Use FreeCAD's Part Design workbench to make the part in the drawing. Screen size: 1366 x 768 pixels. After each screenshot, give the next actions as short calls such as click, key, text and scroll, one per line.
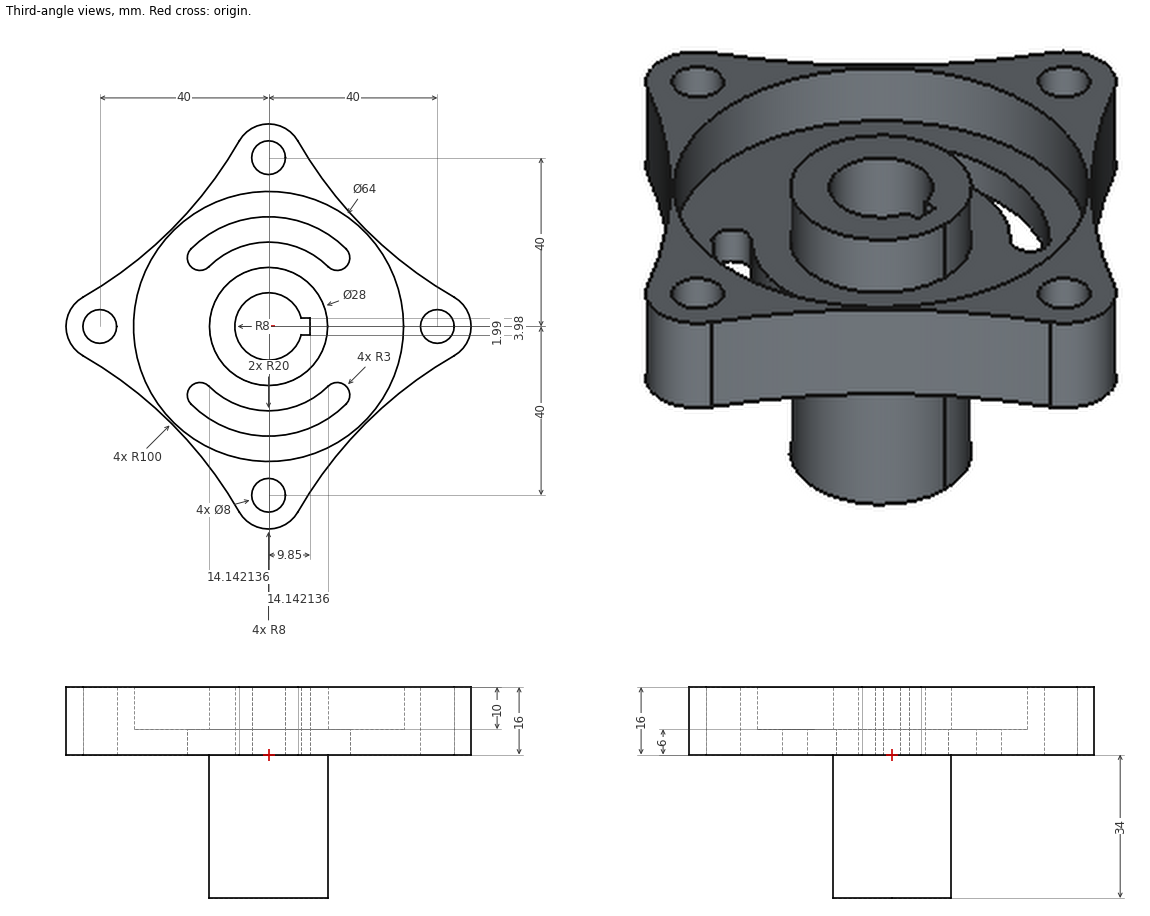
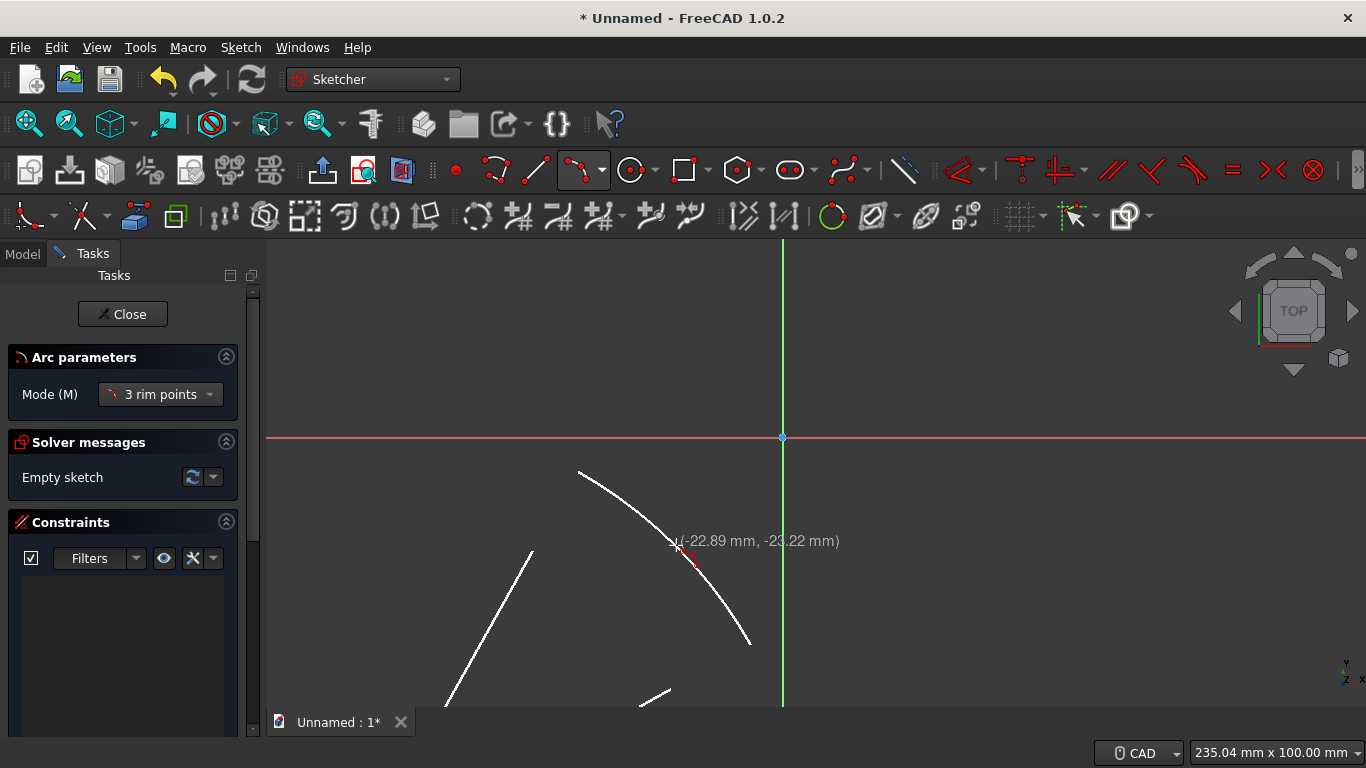
click(675, 545)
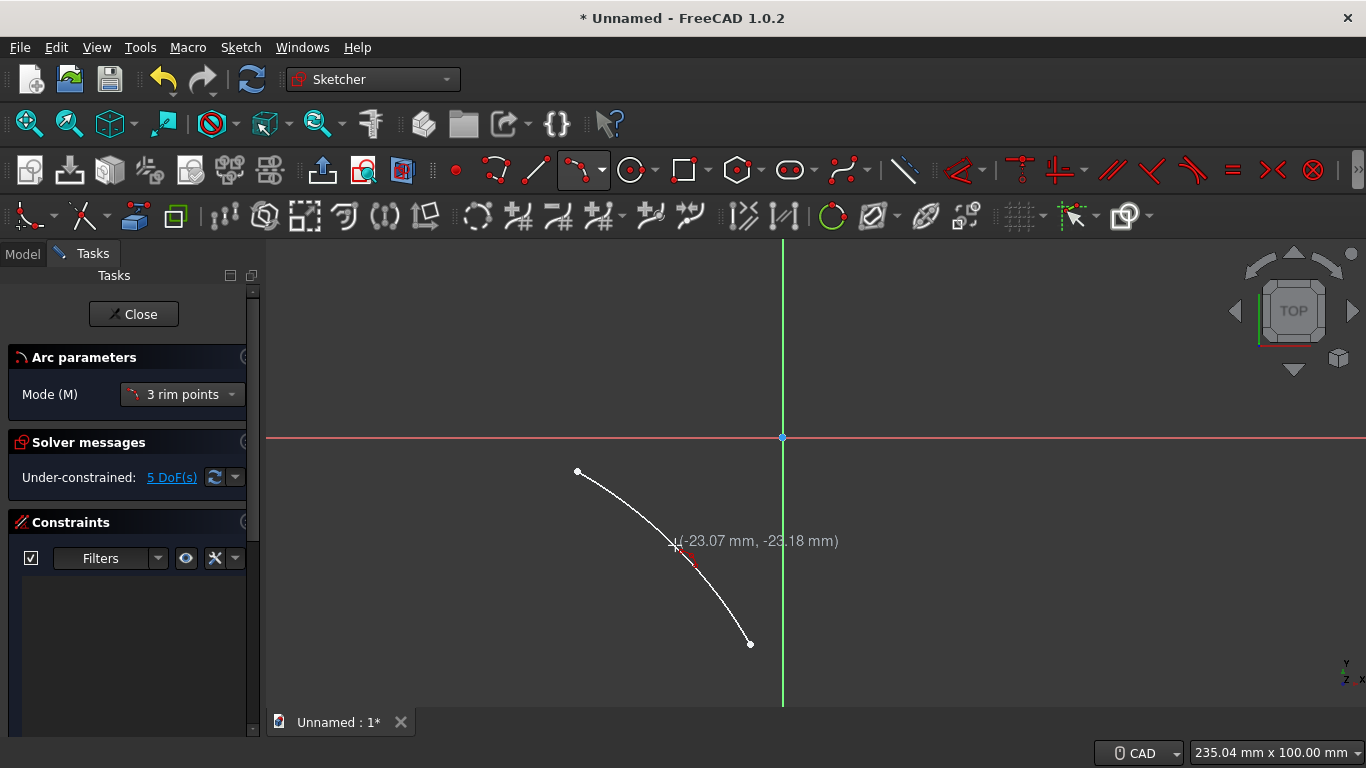
click(750, 645)
click(815, 643)
click(798, 659)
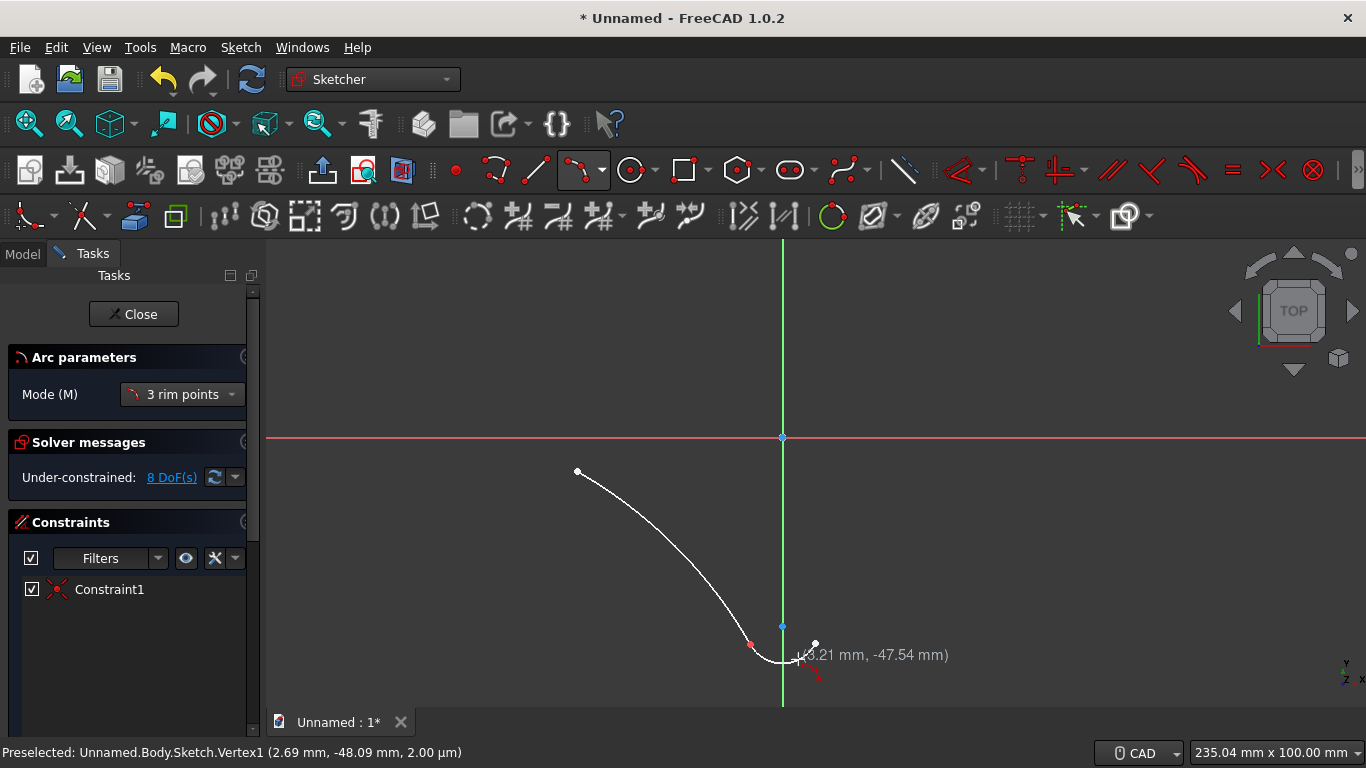
click(815, 644)
click(989, 470)
click(891, 545)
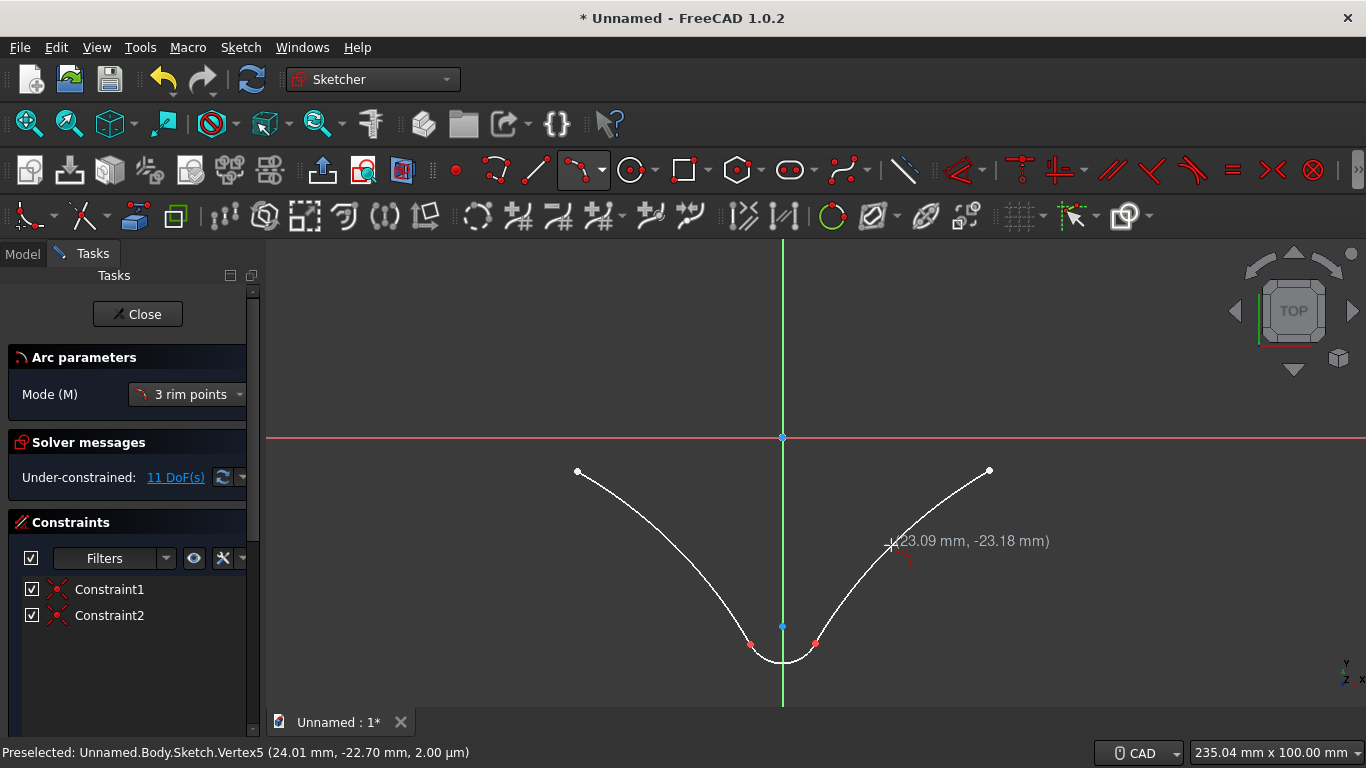
click(989, 471)
click(989, 405)
click(1004, 453)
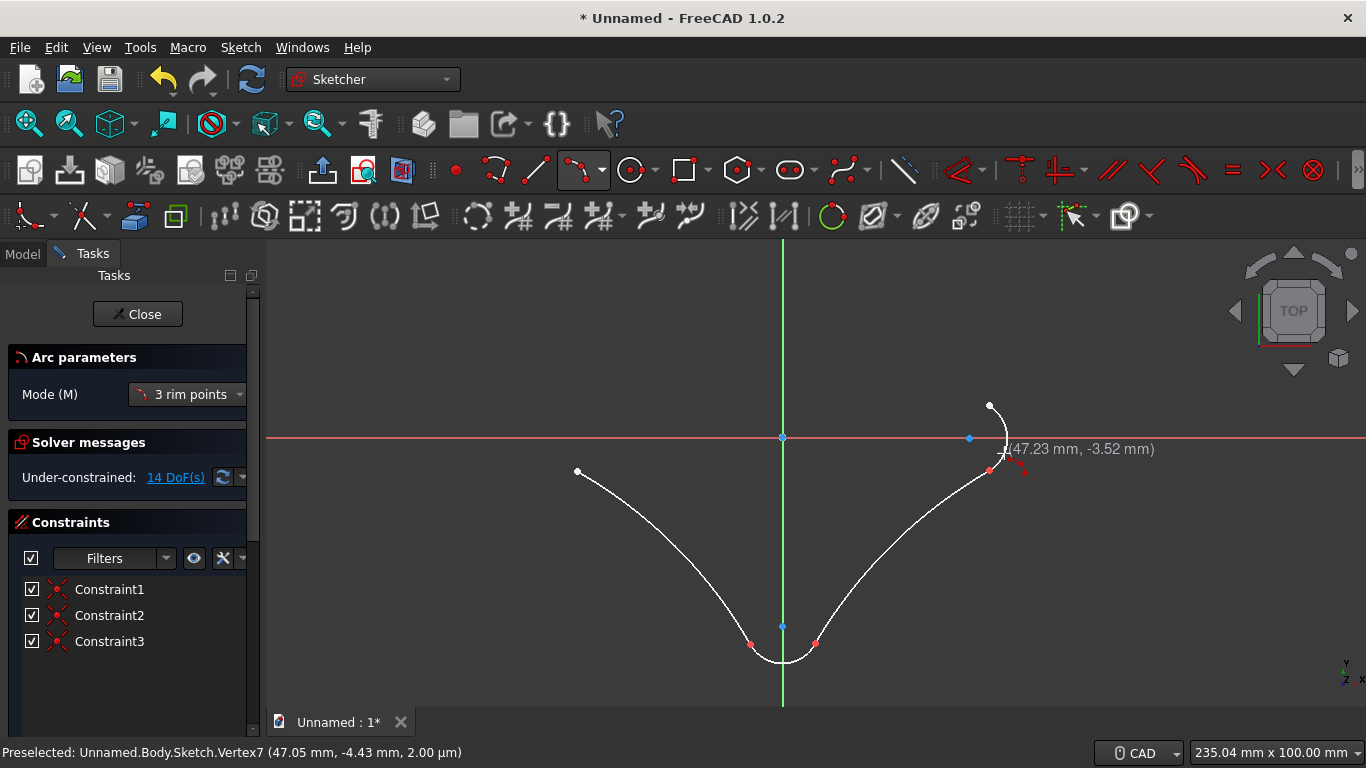
click(989, 406)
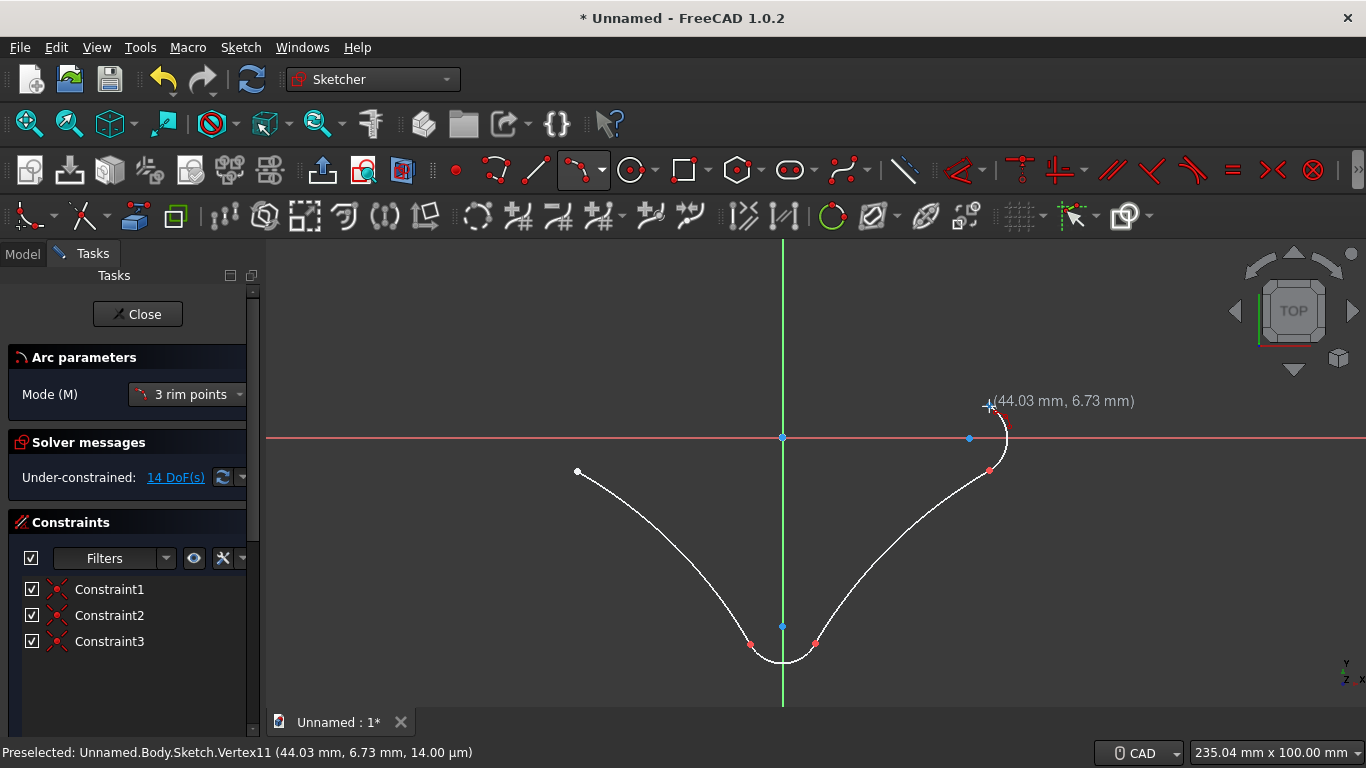
scroll(675, 545, down, 2)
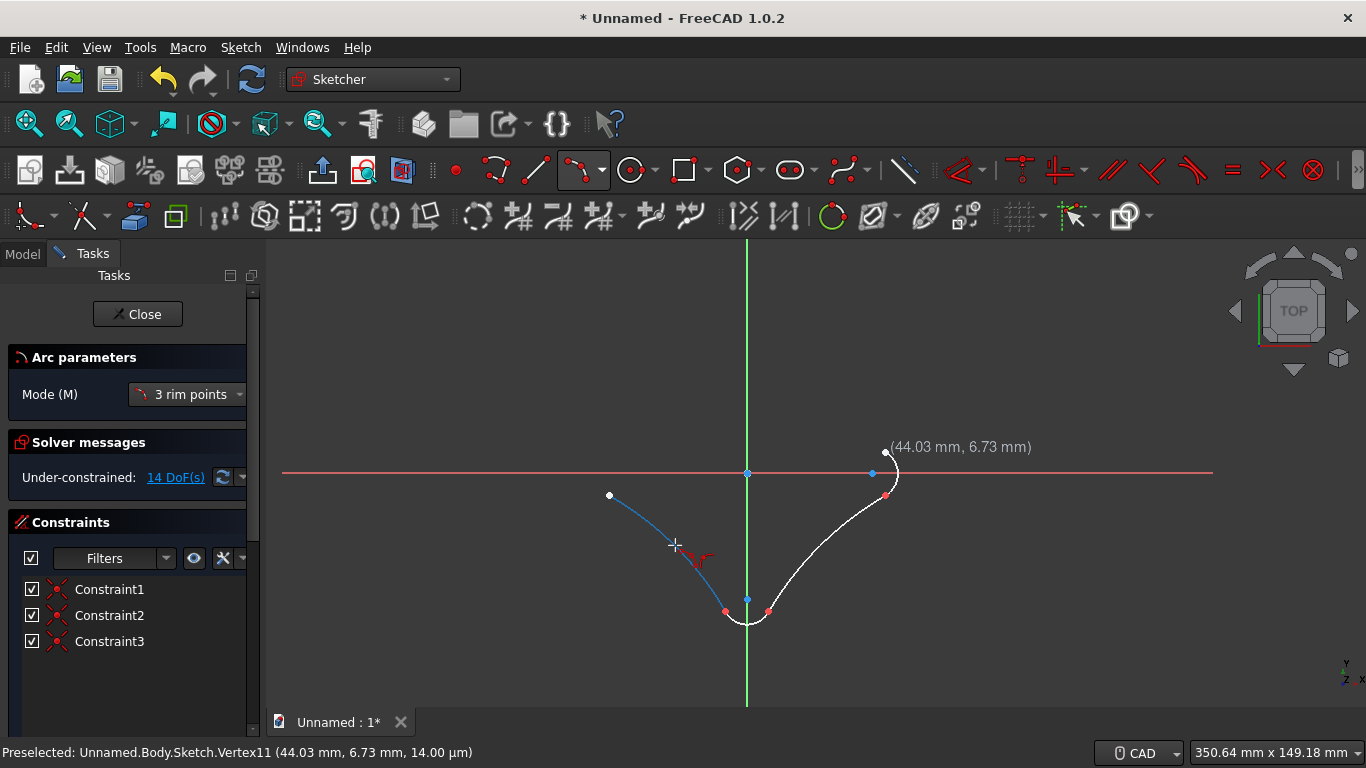
click(769, 335)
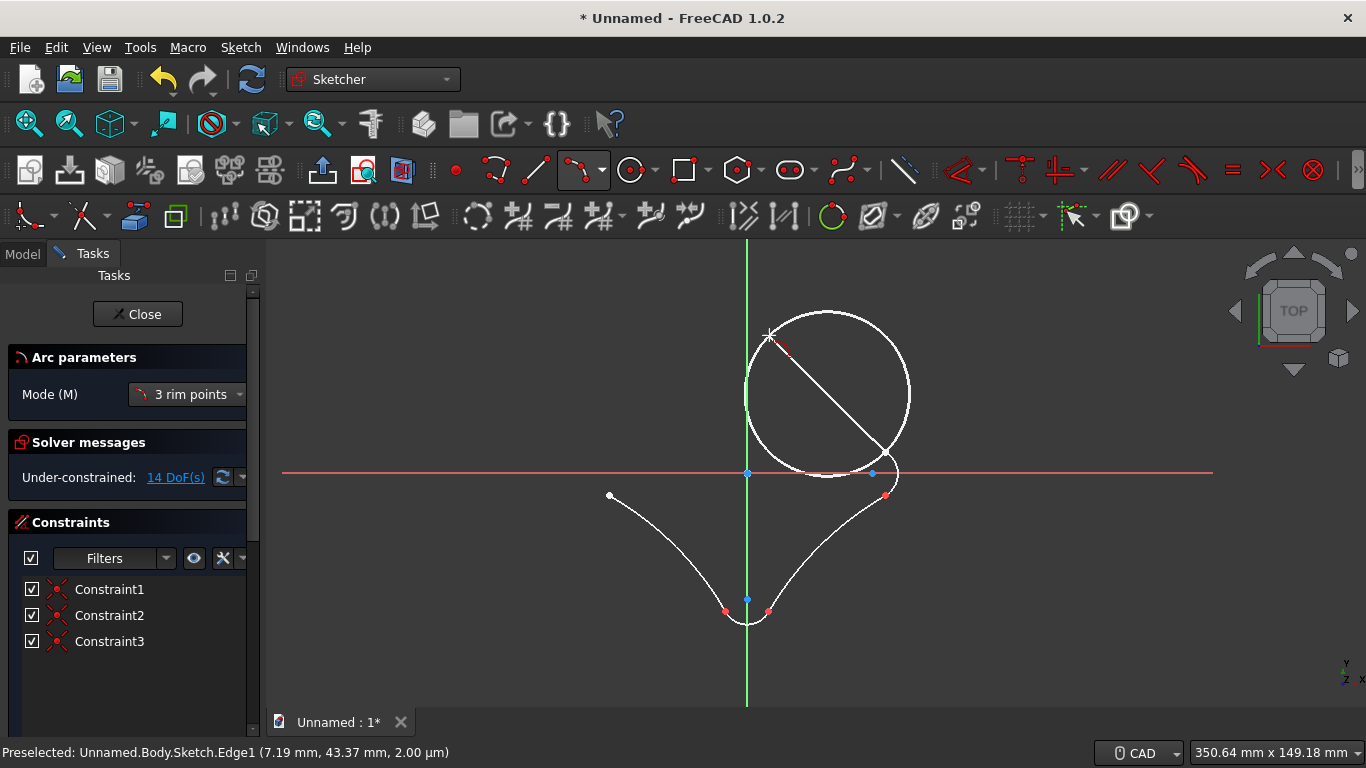
scroll(820, 401, up, 2)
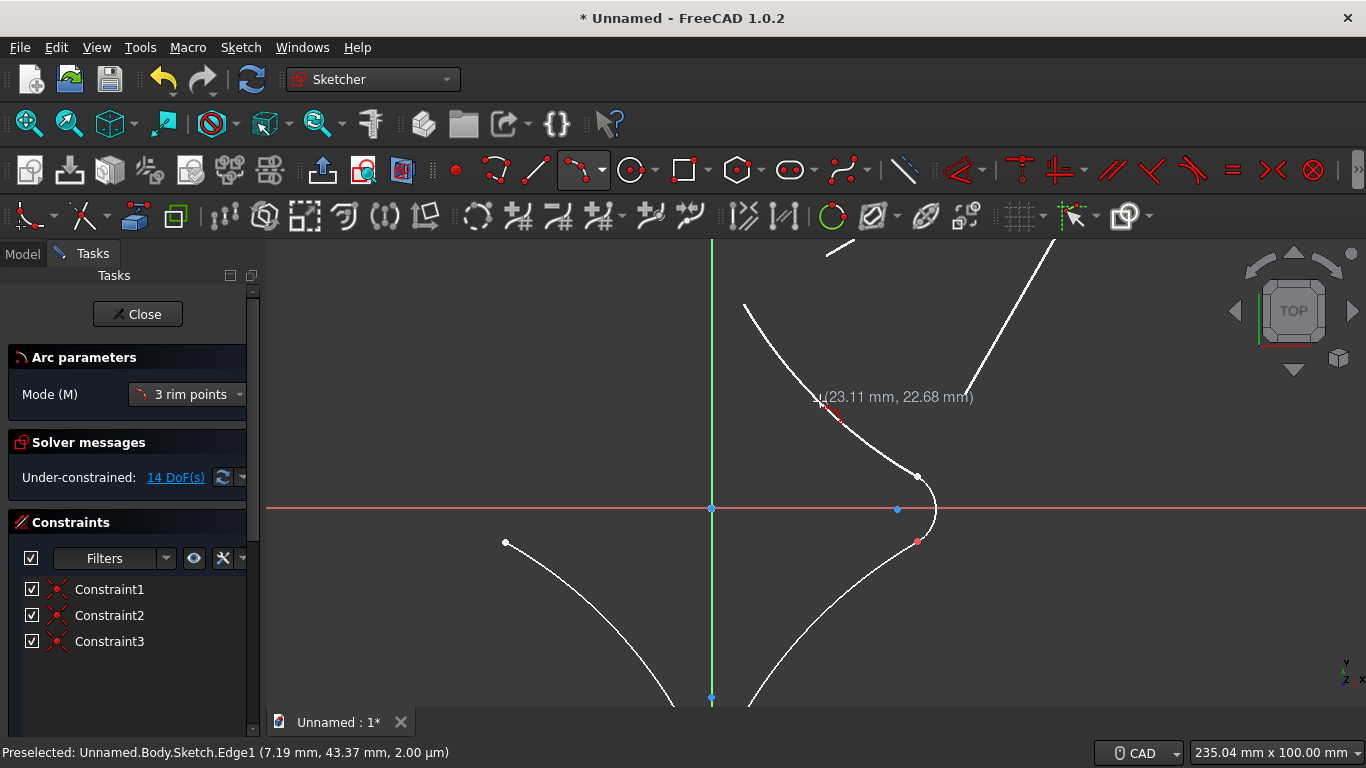
click(819, 401)